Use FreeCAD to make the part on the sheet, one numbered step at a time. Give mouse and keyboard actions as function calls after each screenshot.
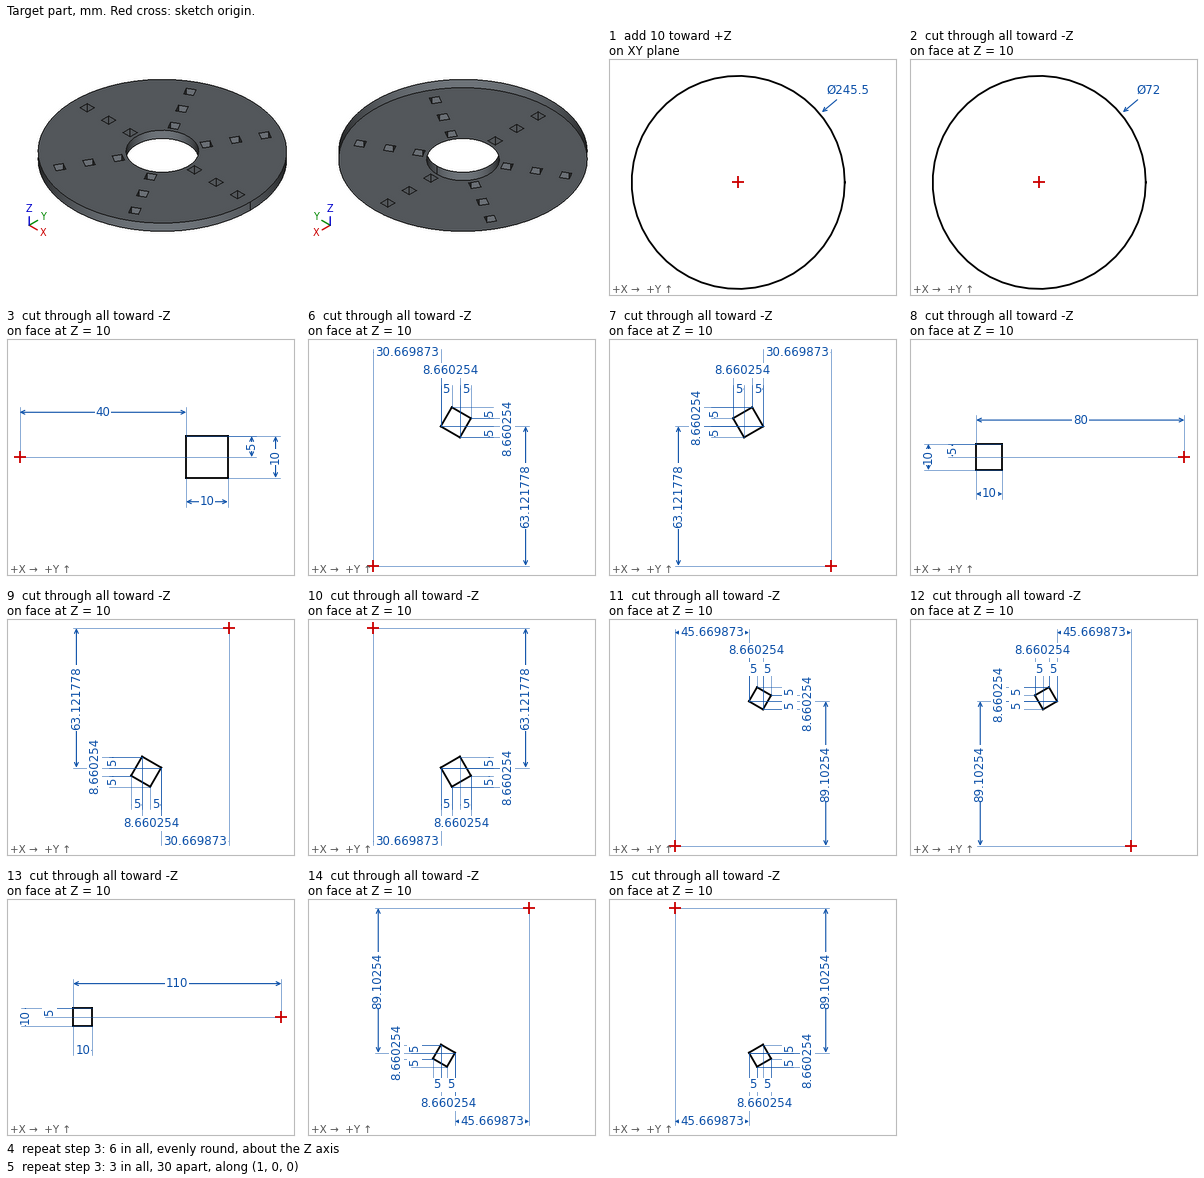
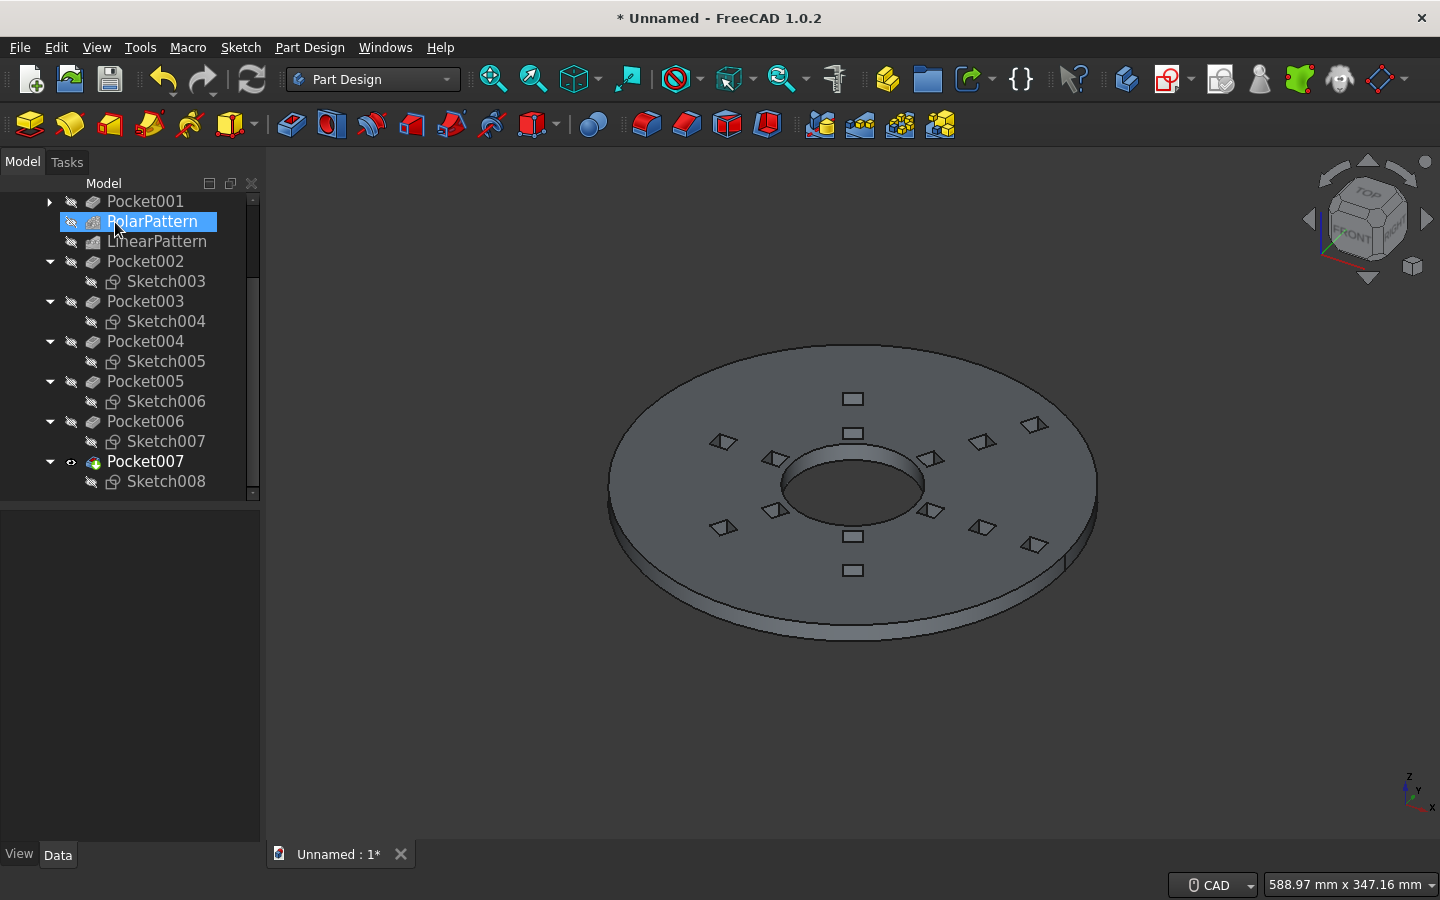
click(923, 414)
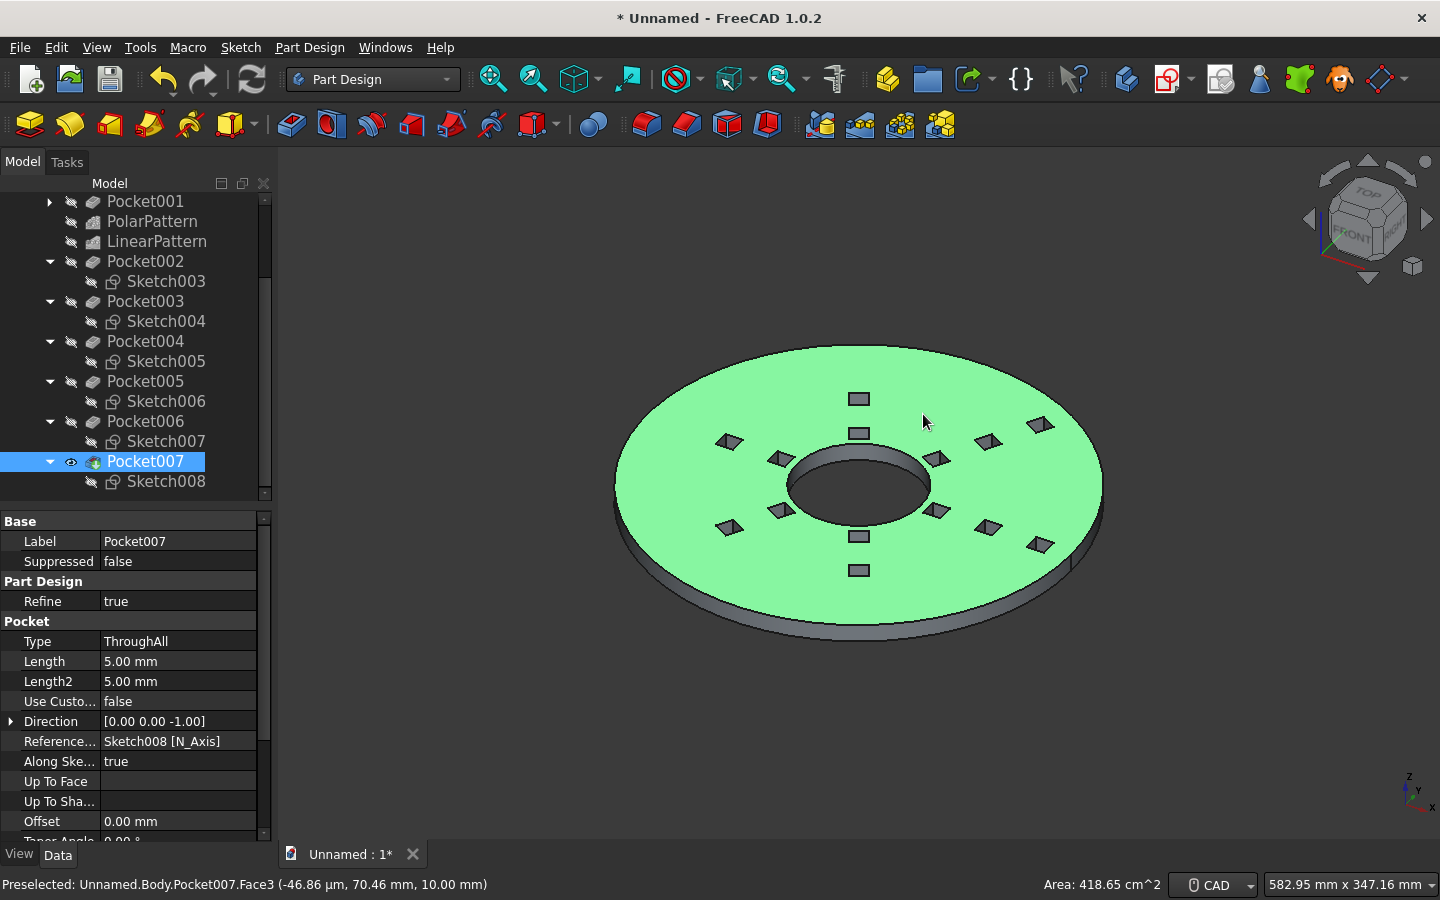
click(1168, 80)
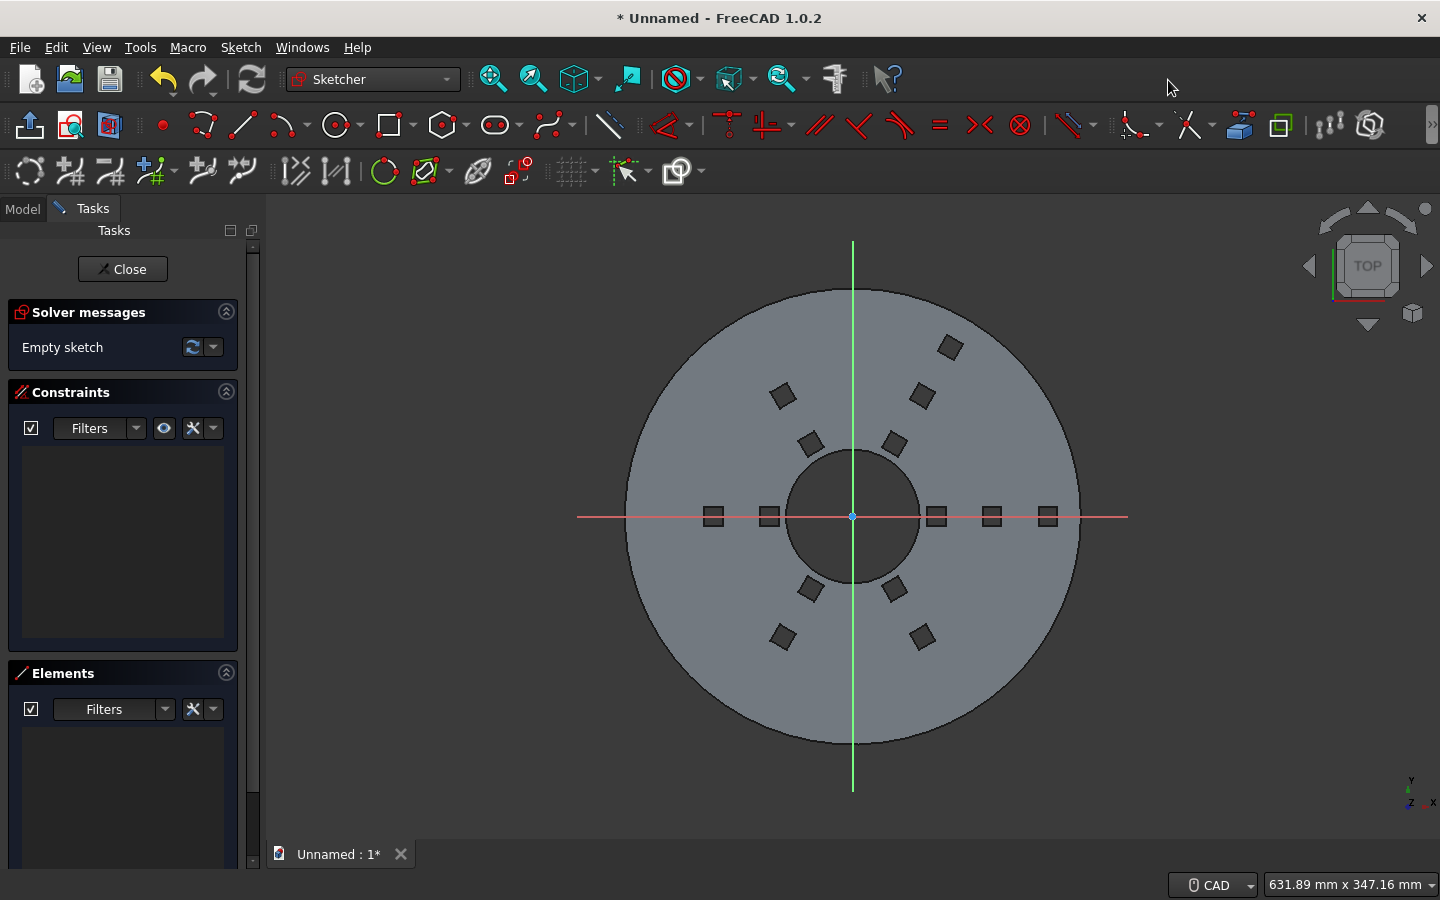
scroll(753, 337, up, 14)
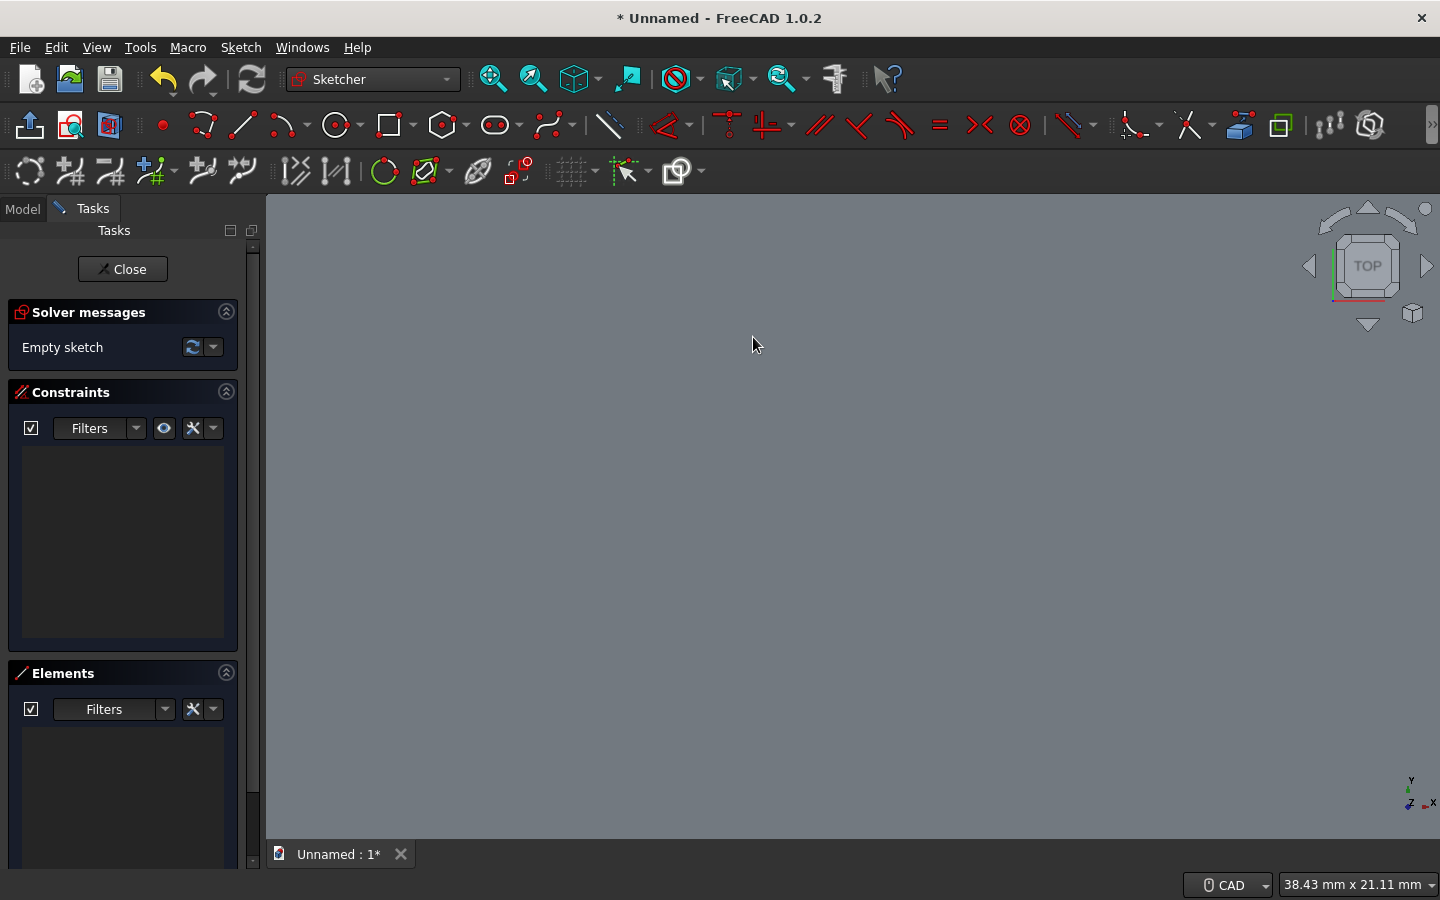
click(204, 126)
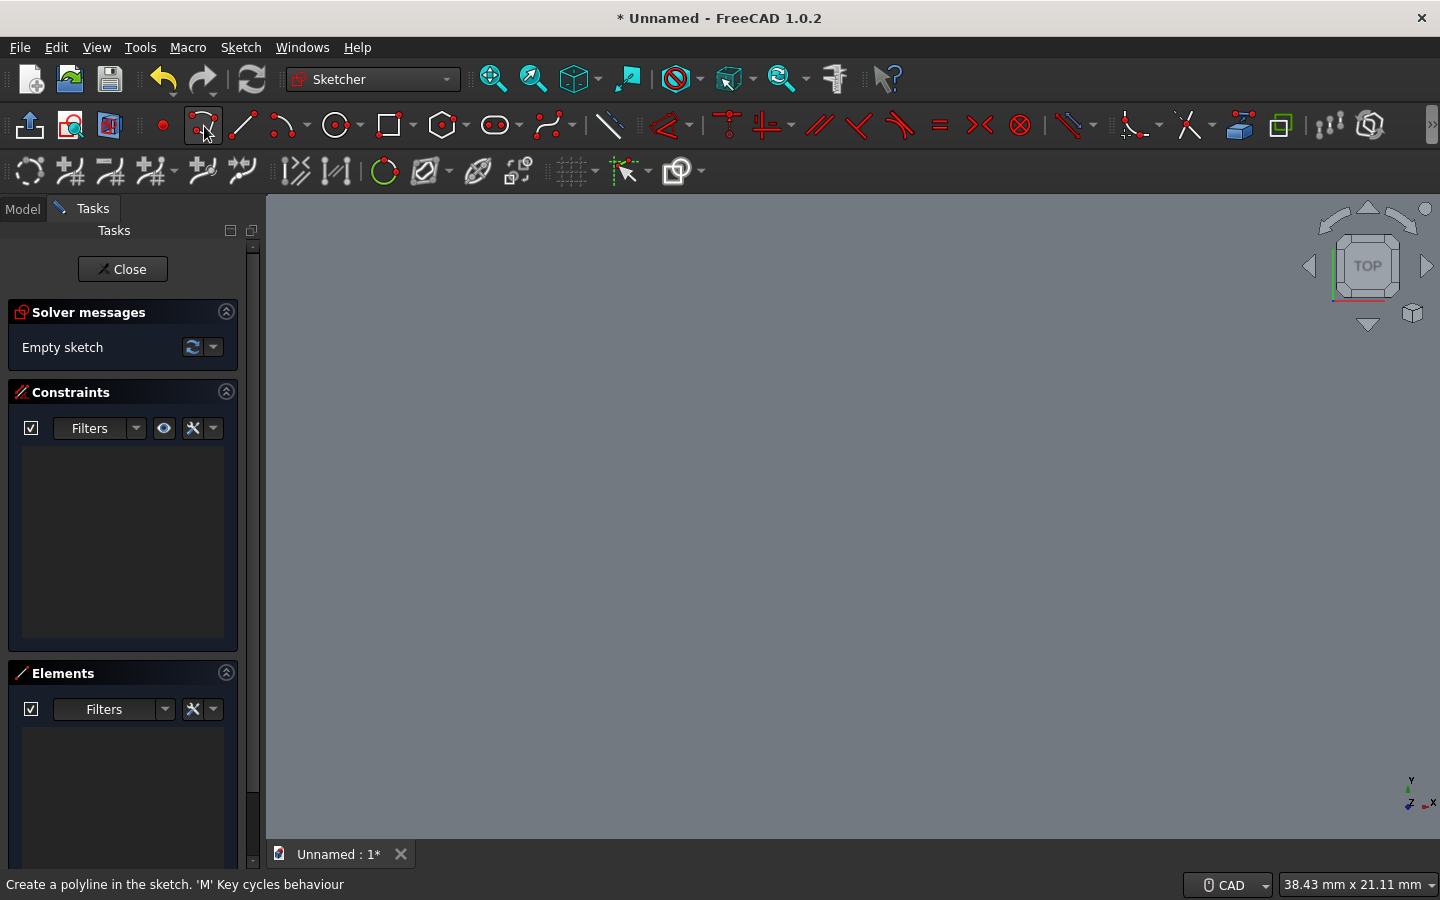
click(993, 563)
click(840, 298)
click(576, 451)
click(729, 716)
click(993, 564)
key(Escape)
key(Escape)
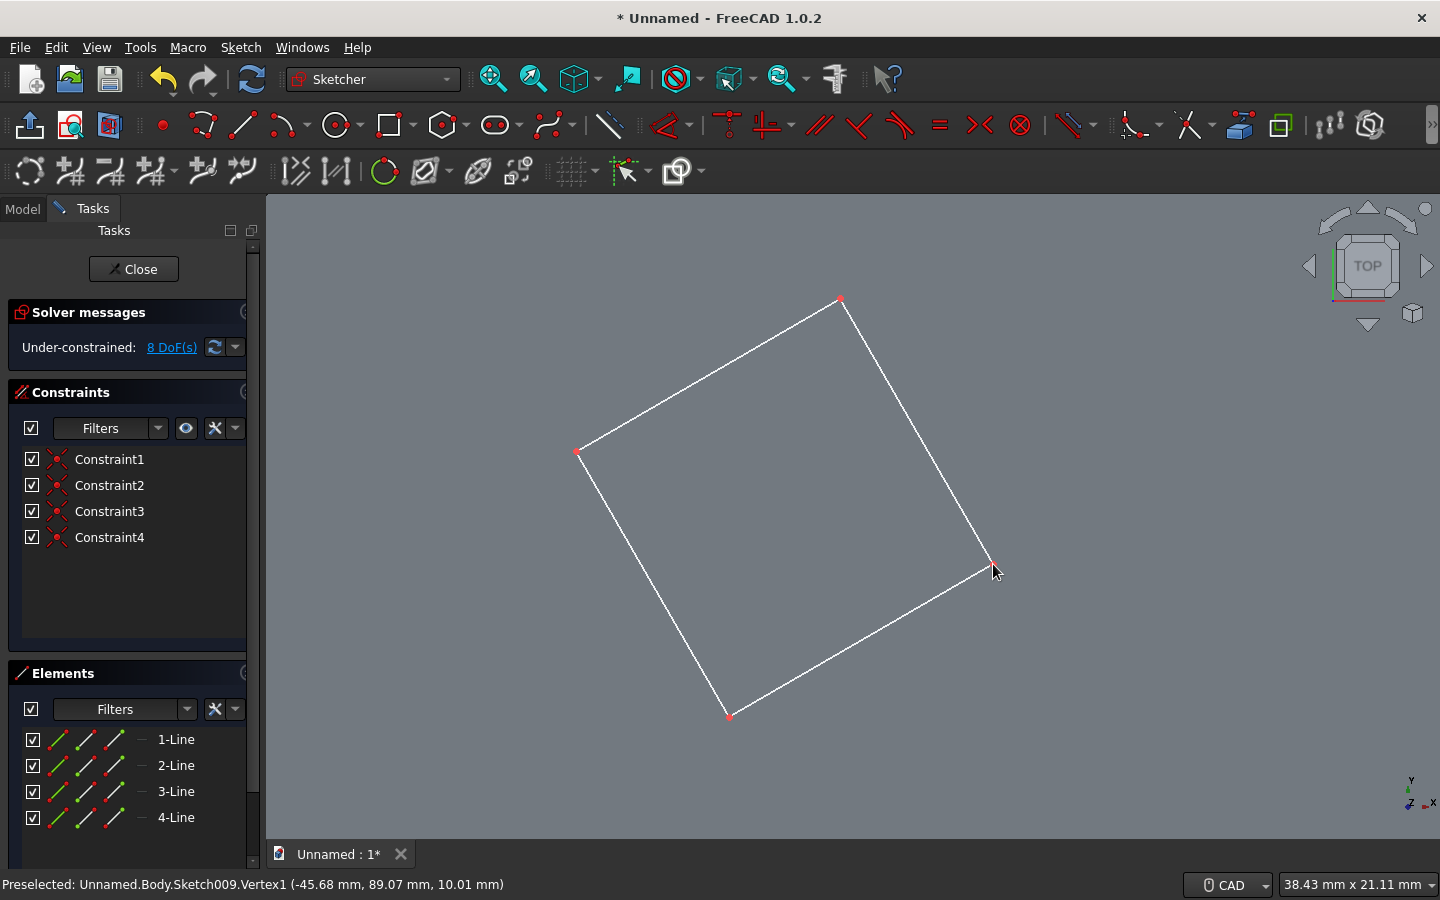
click(664, 126)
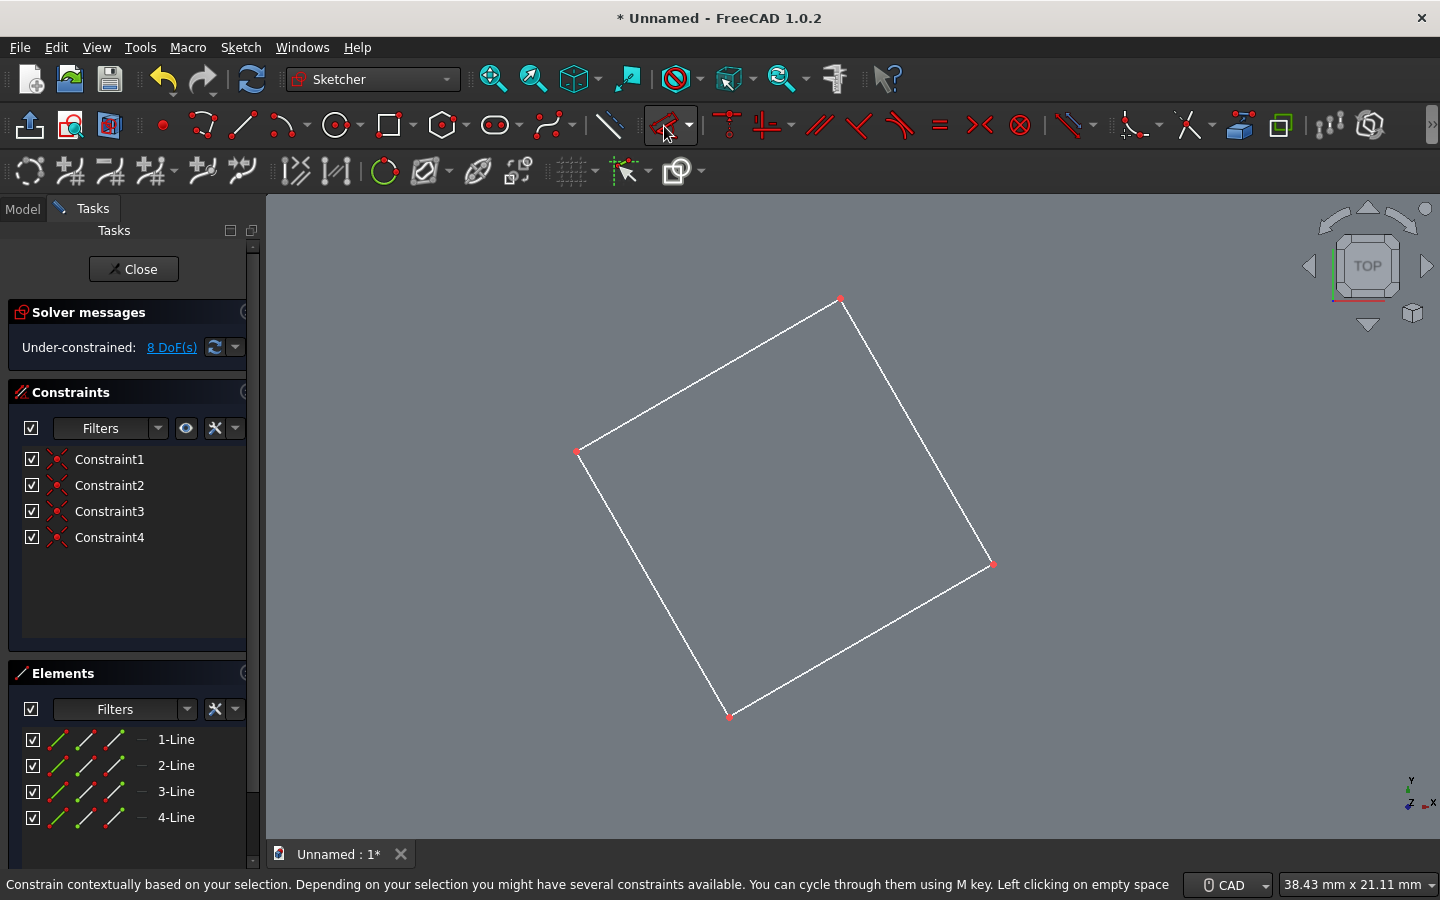
click(947, 485)
click(916, 265)